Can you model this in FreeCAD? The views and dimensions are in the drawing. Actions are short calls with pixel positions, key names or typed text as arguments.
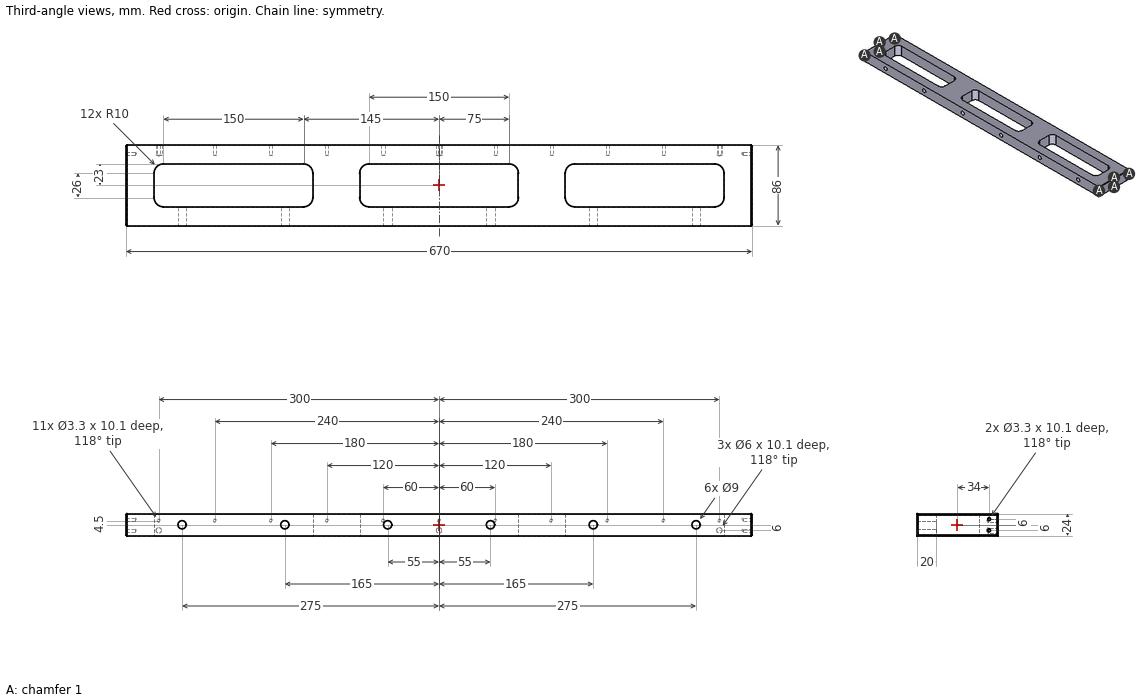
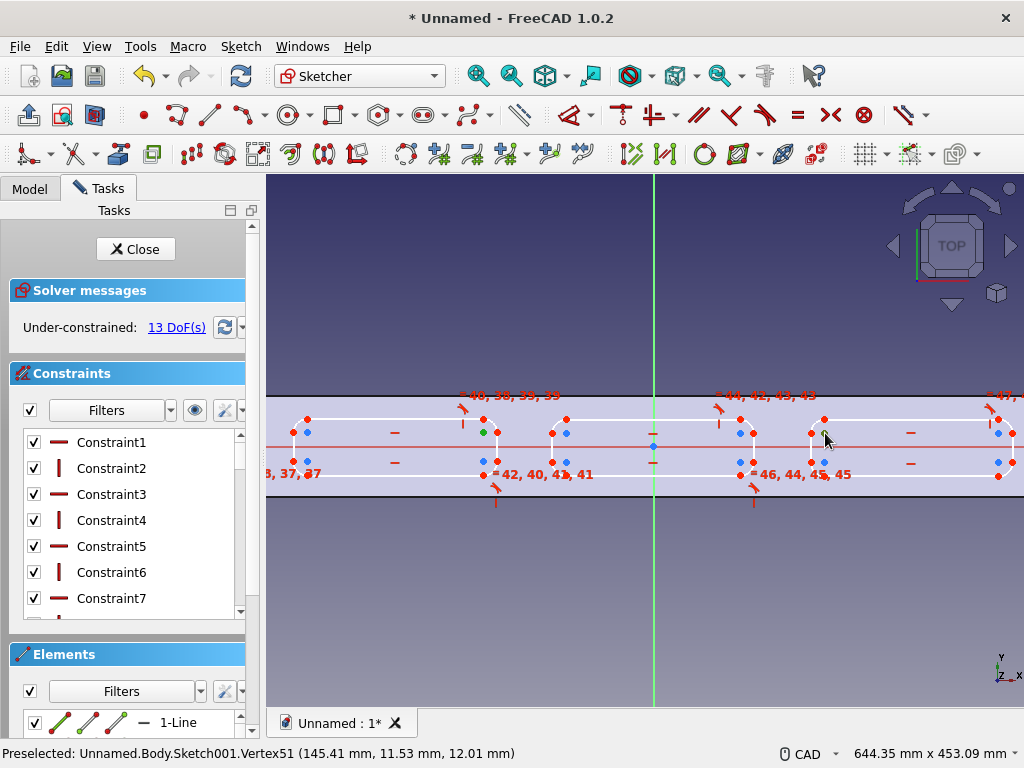
click(654, 645)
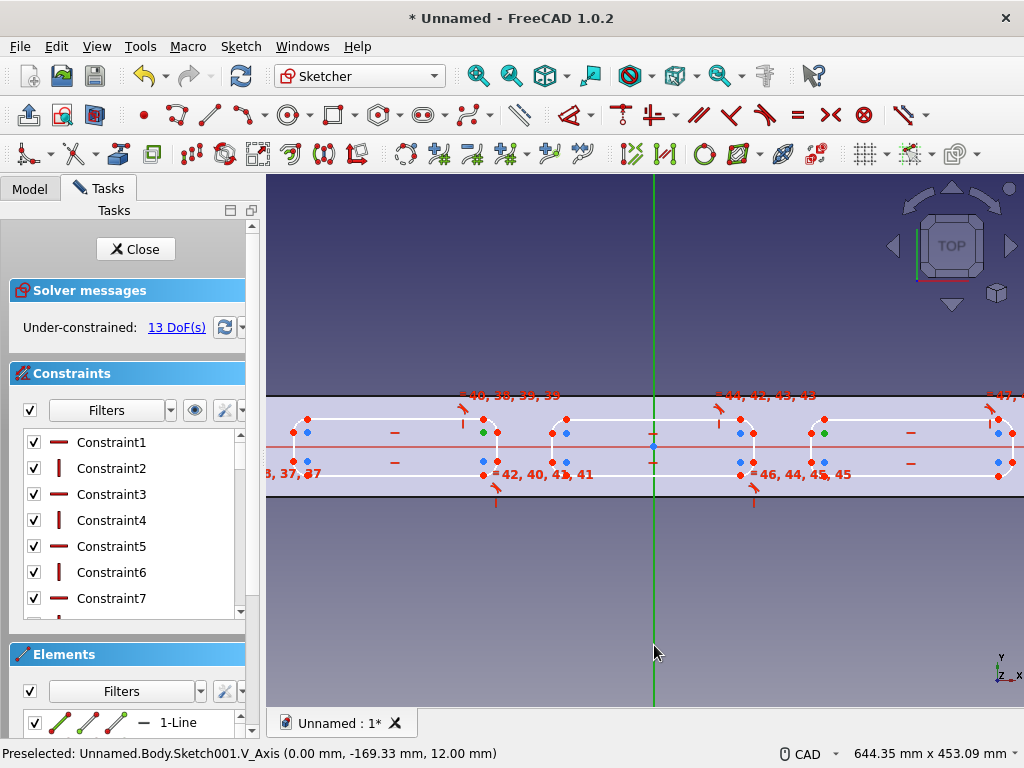
key(s)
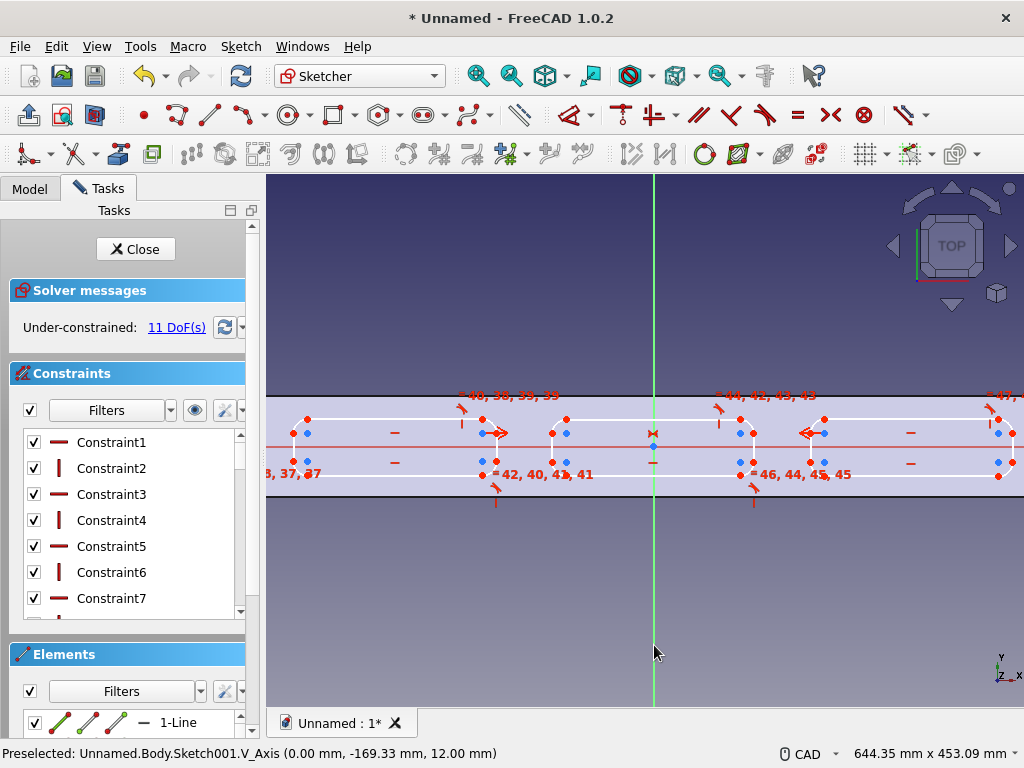
click(307, 462)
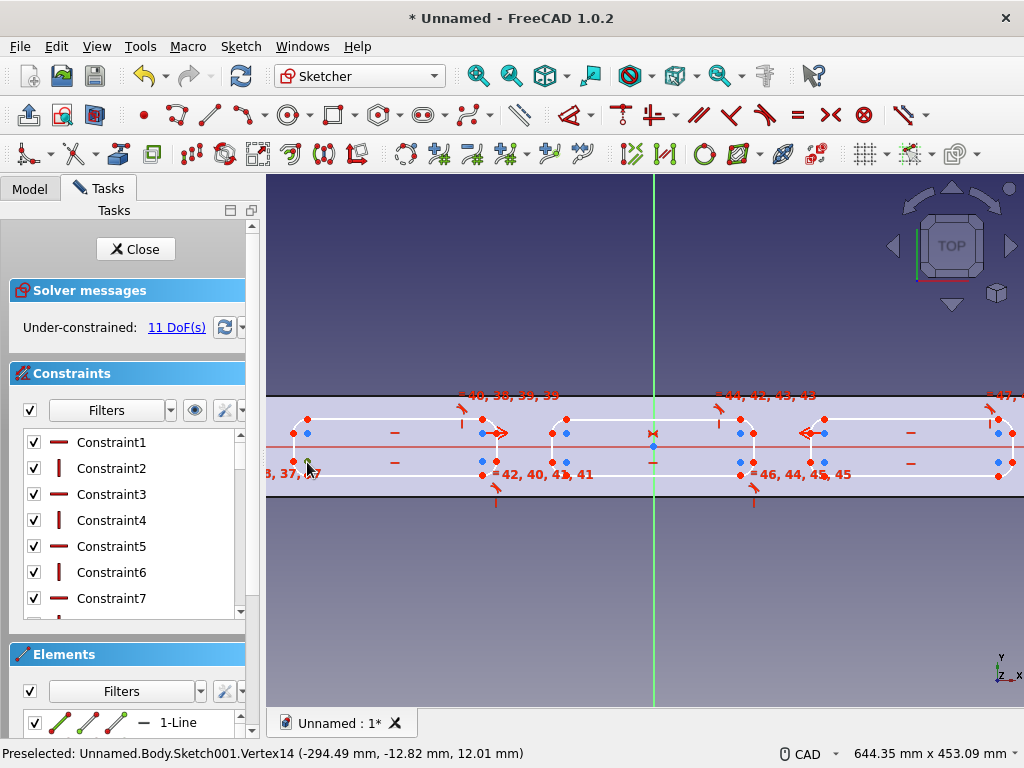
scroll(483, 433, down, 3)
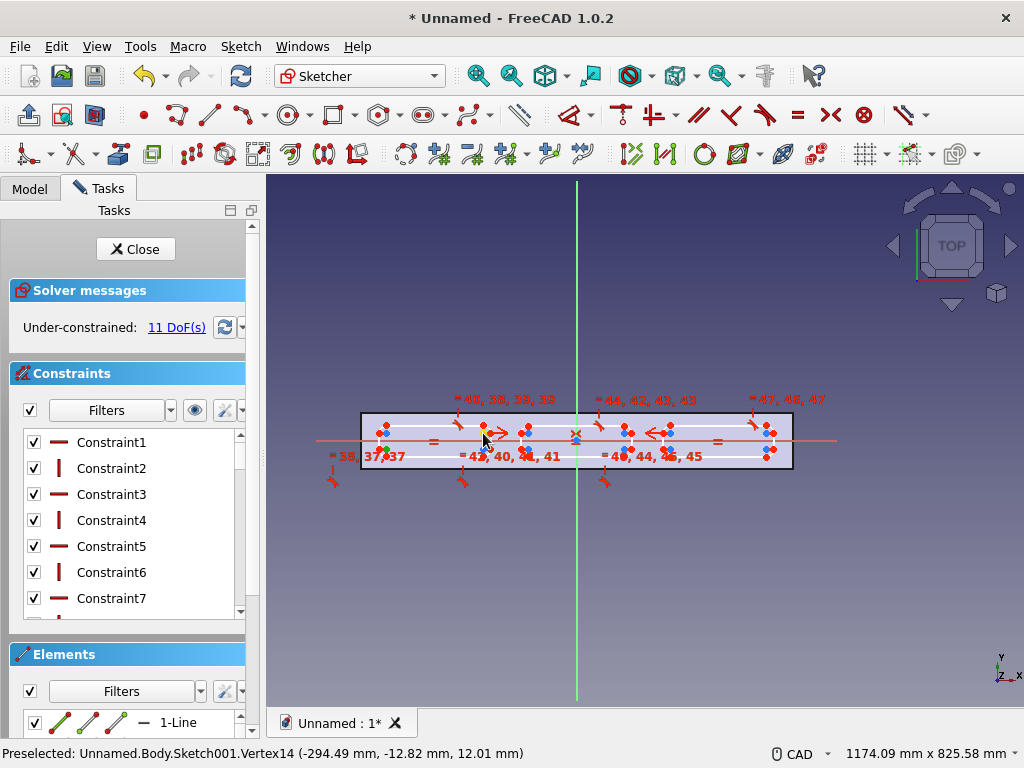
scroll(766, 449, up, 3)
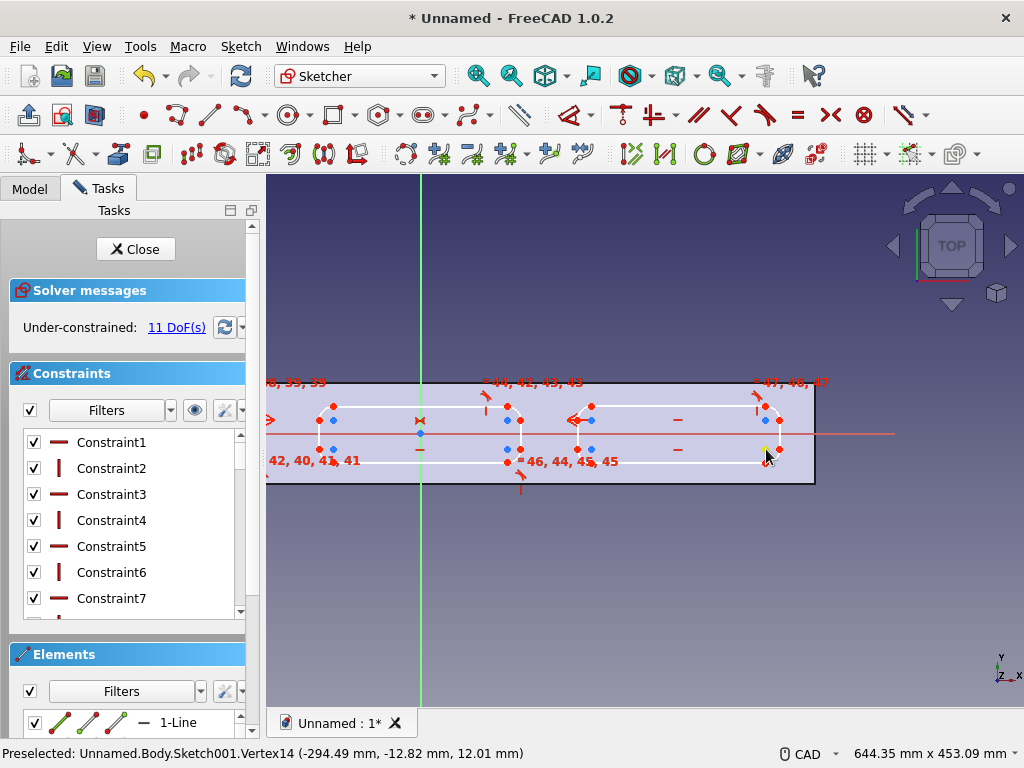
click(766, 449)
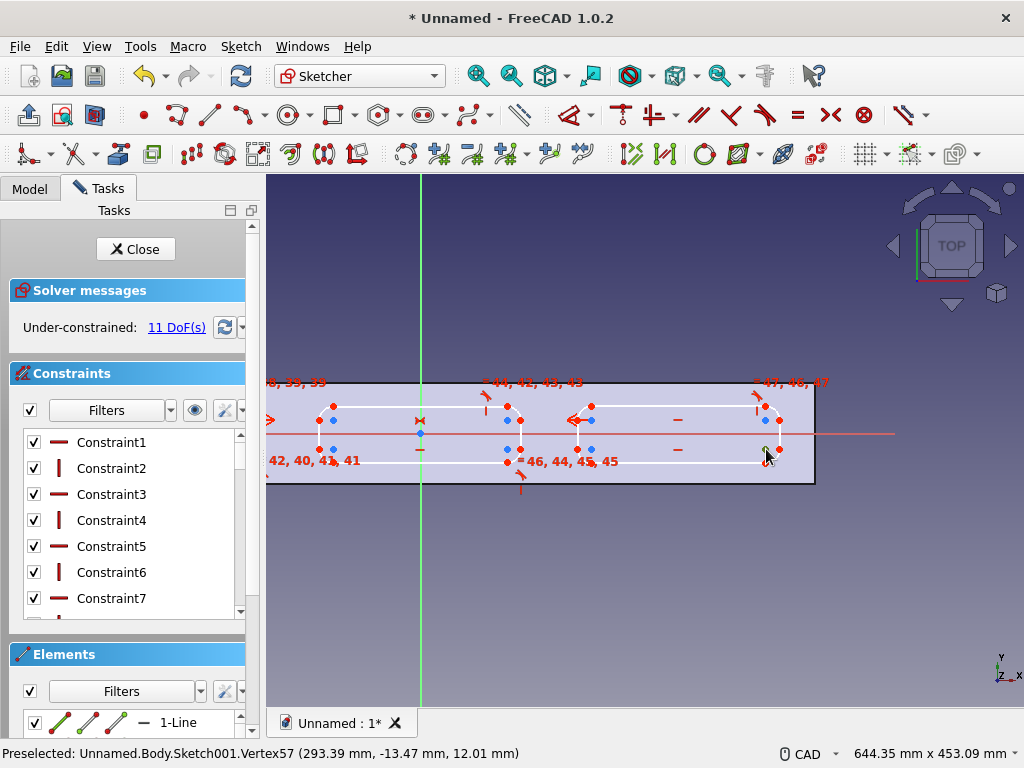
click(421, 645)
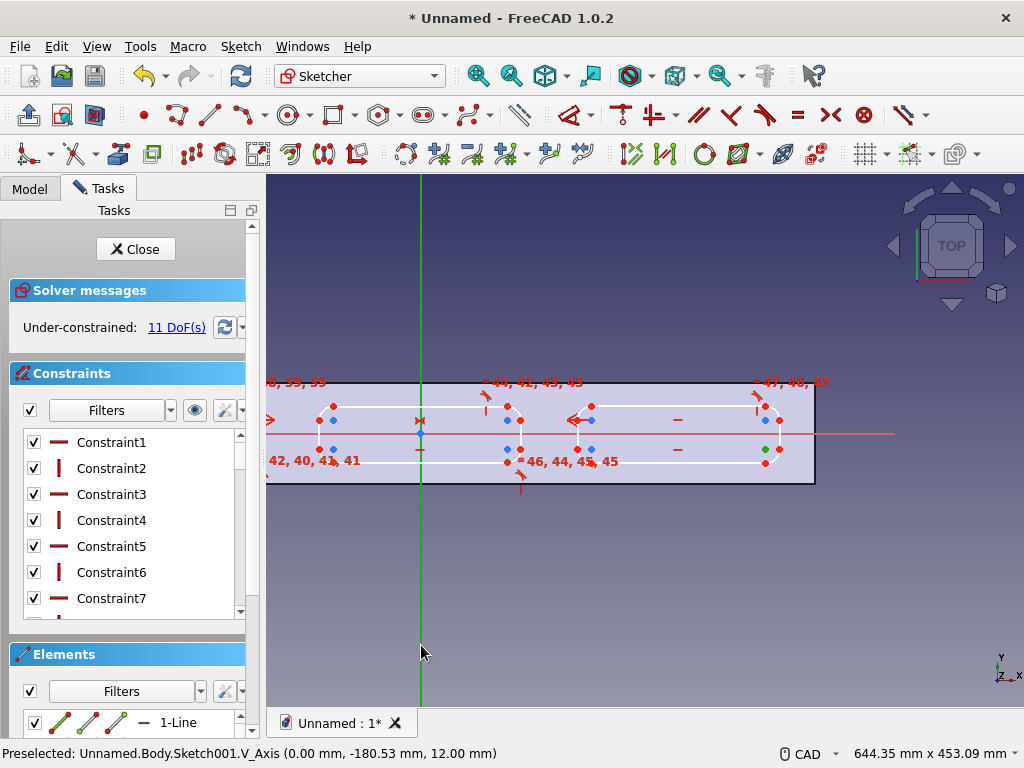
key(s)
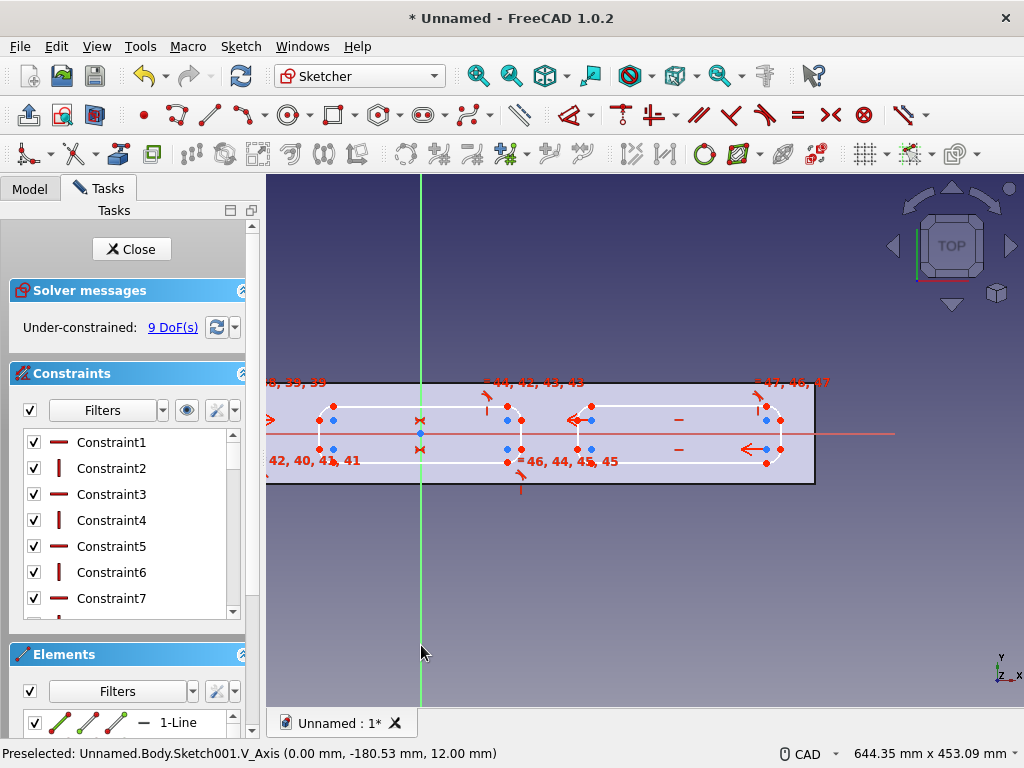
click(568, 116)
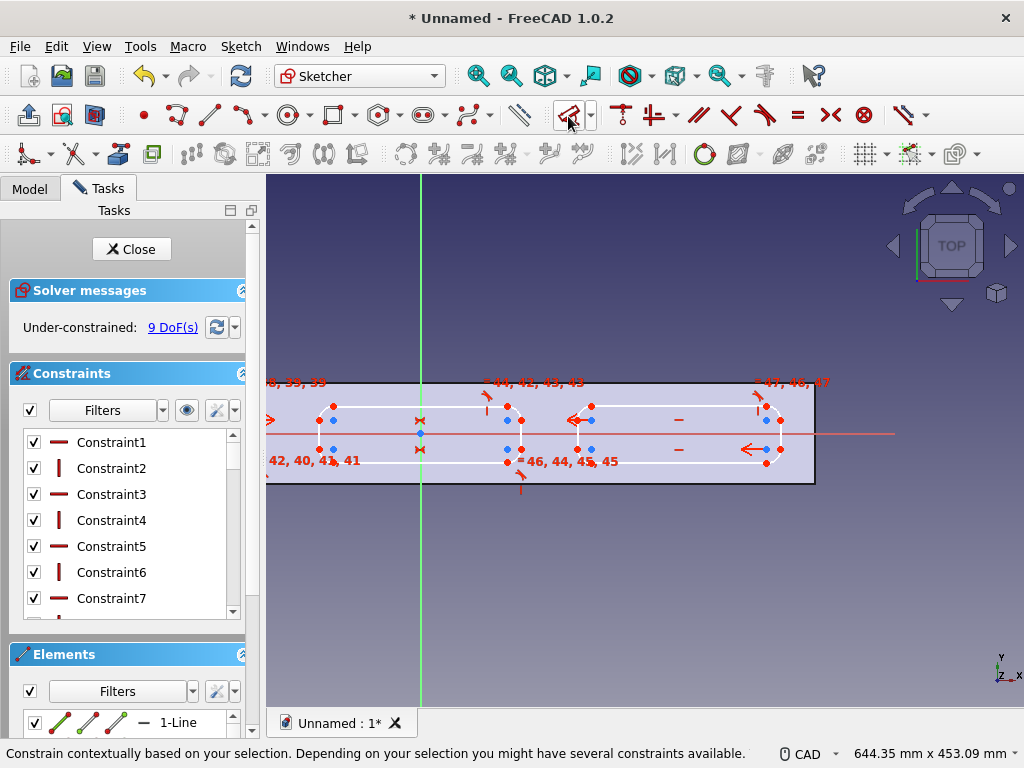
scroll(766, 449, down, 3)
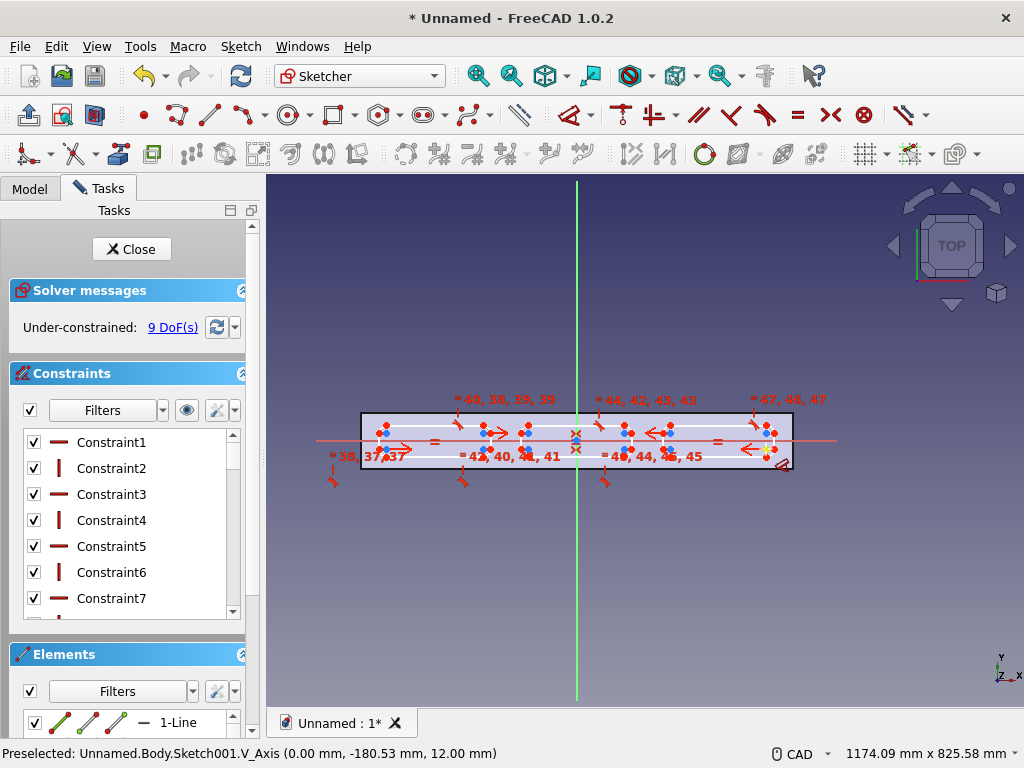
scroll(382, 428, up, 10)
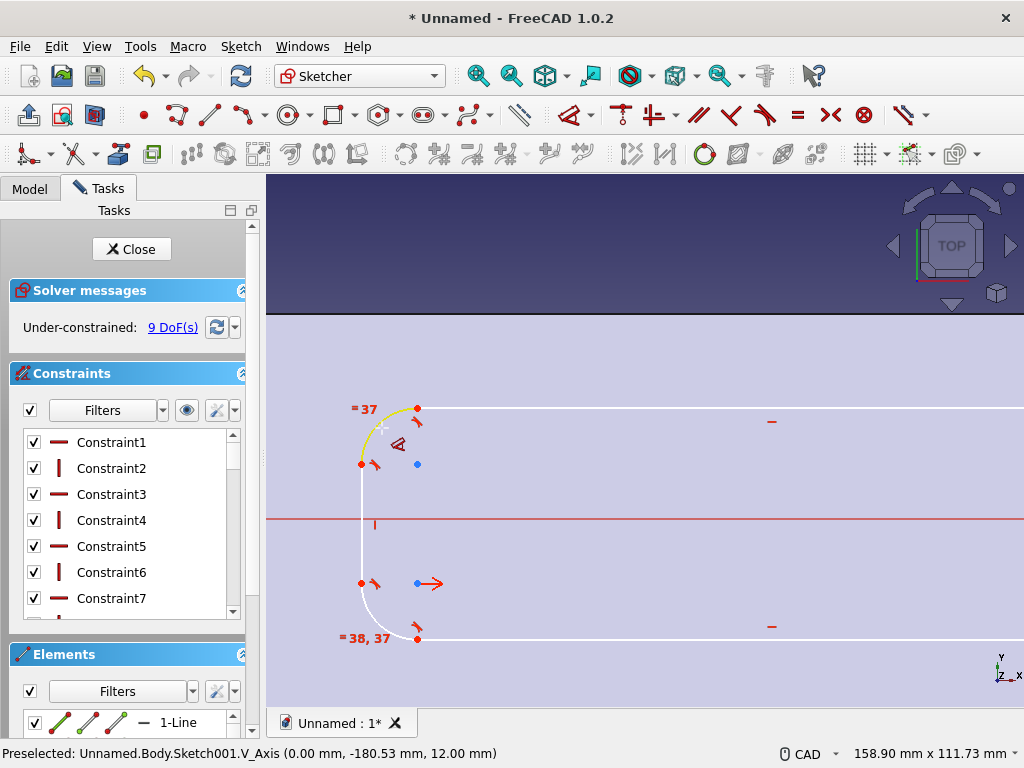
click(378, 425)
click(355, 402)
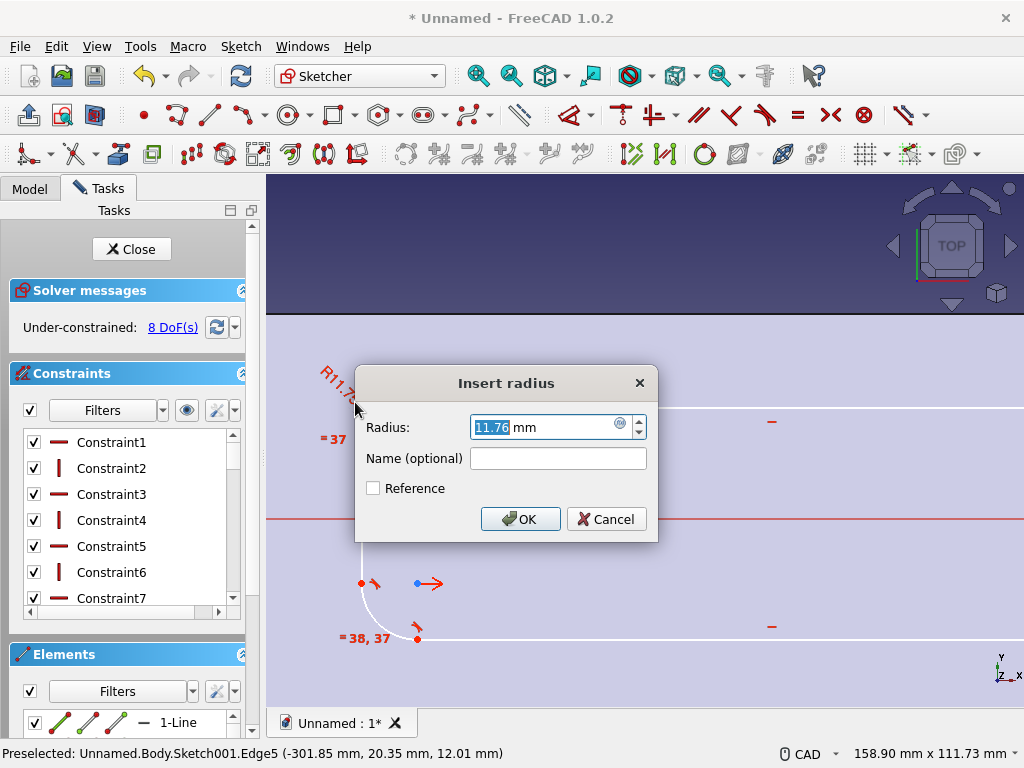
text(10)
key(Return)